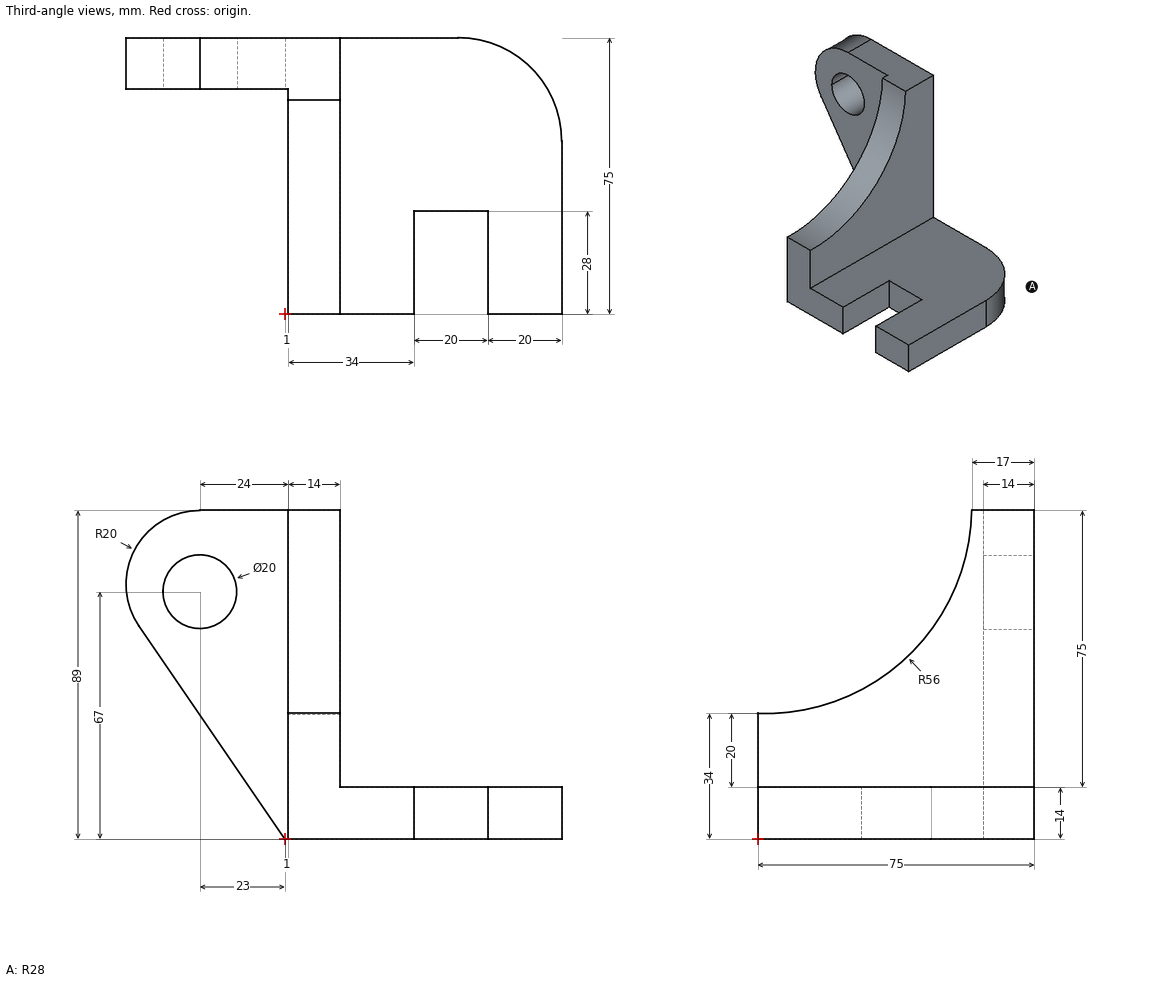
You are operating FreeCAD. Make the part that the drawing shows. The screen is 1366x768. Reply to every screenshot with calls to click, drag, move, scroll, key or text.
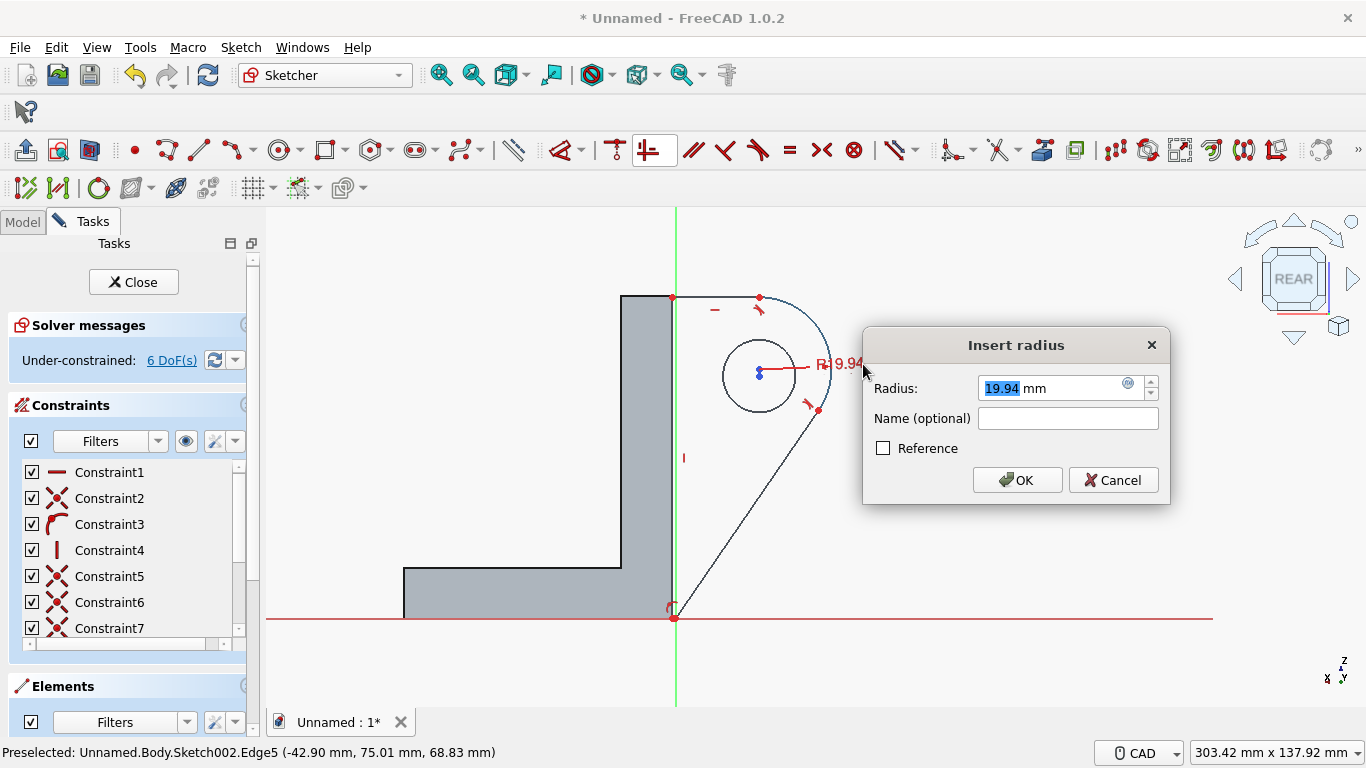
text(20)
key(Return)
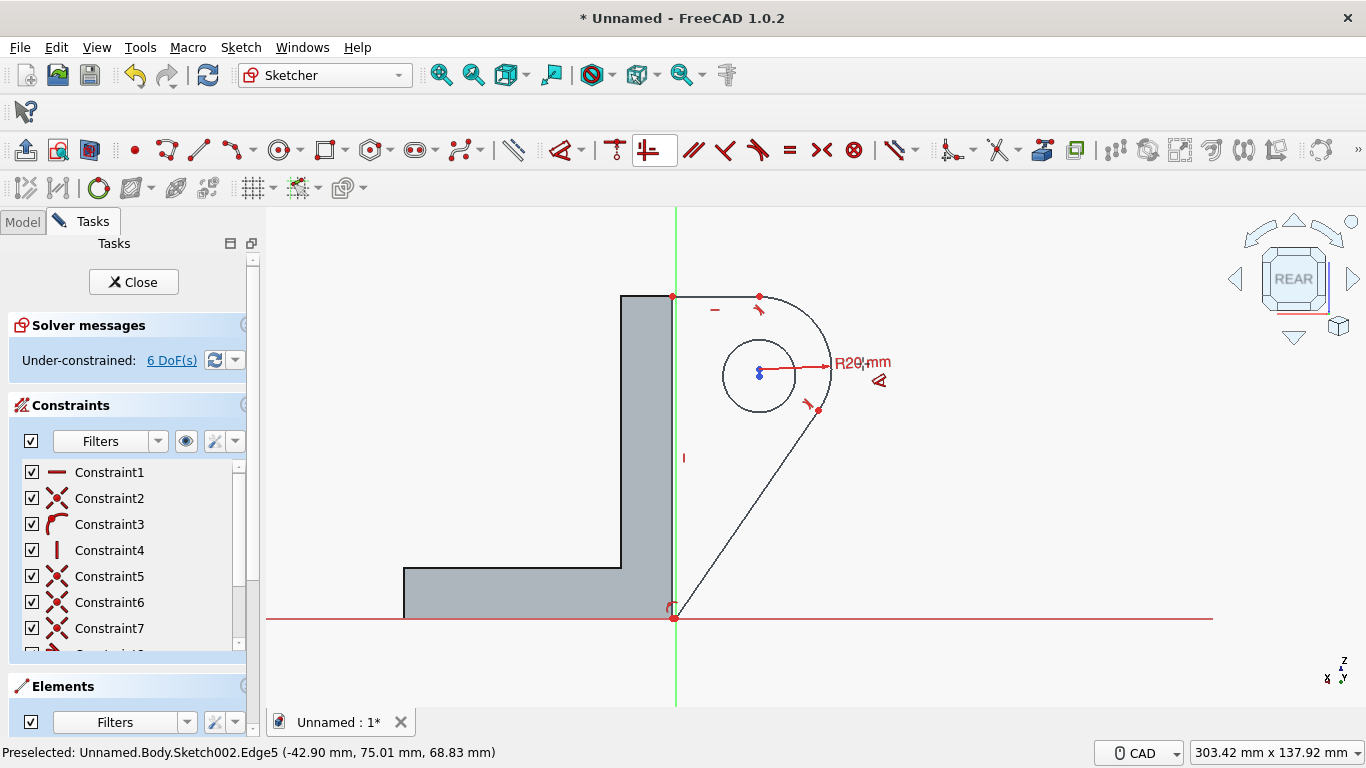
click(785, 350)
click(710, 328)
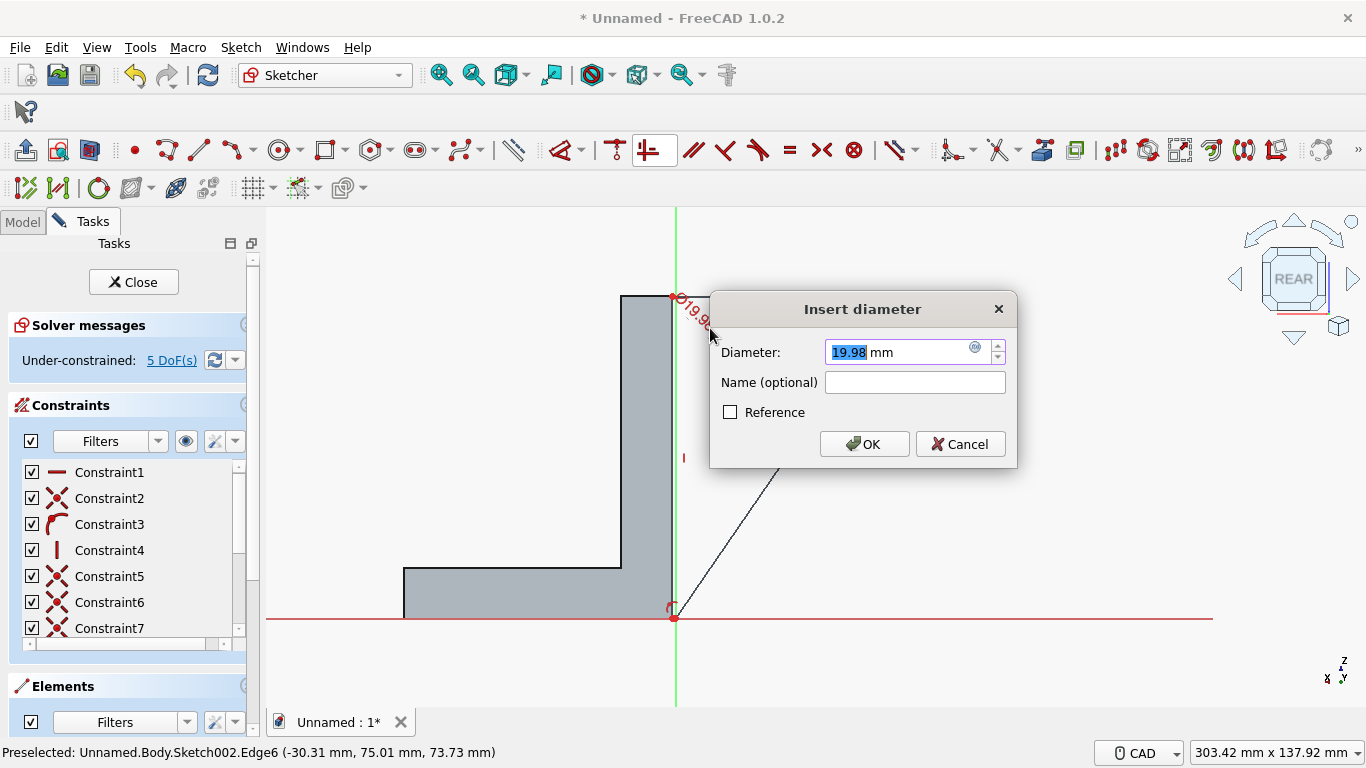
text(20)
key(Return)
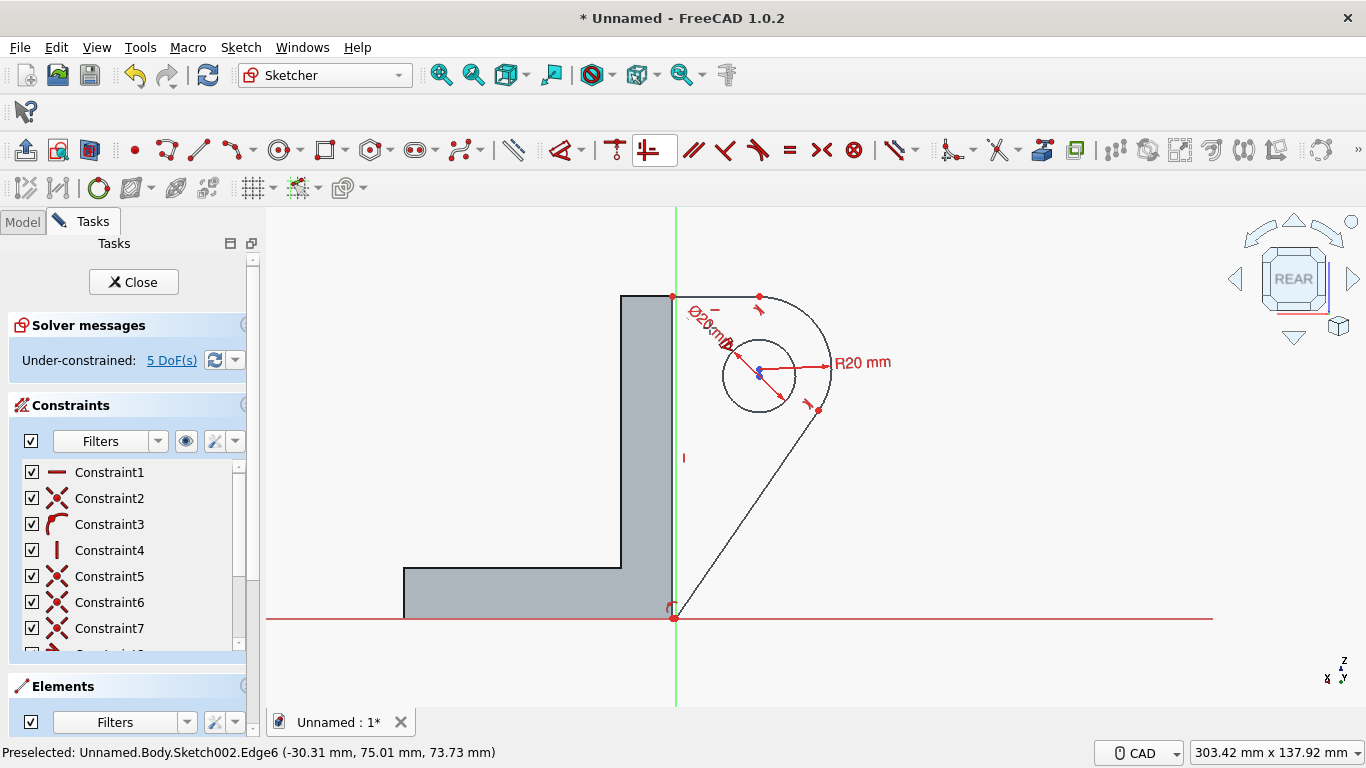
scroll(674, 619, up, 12)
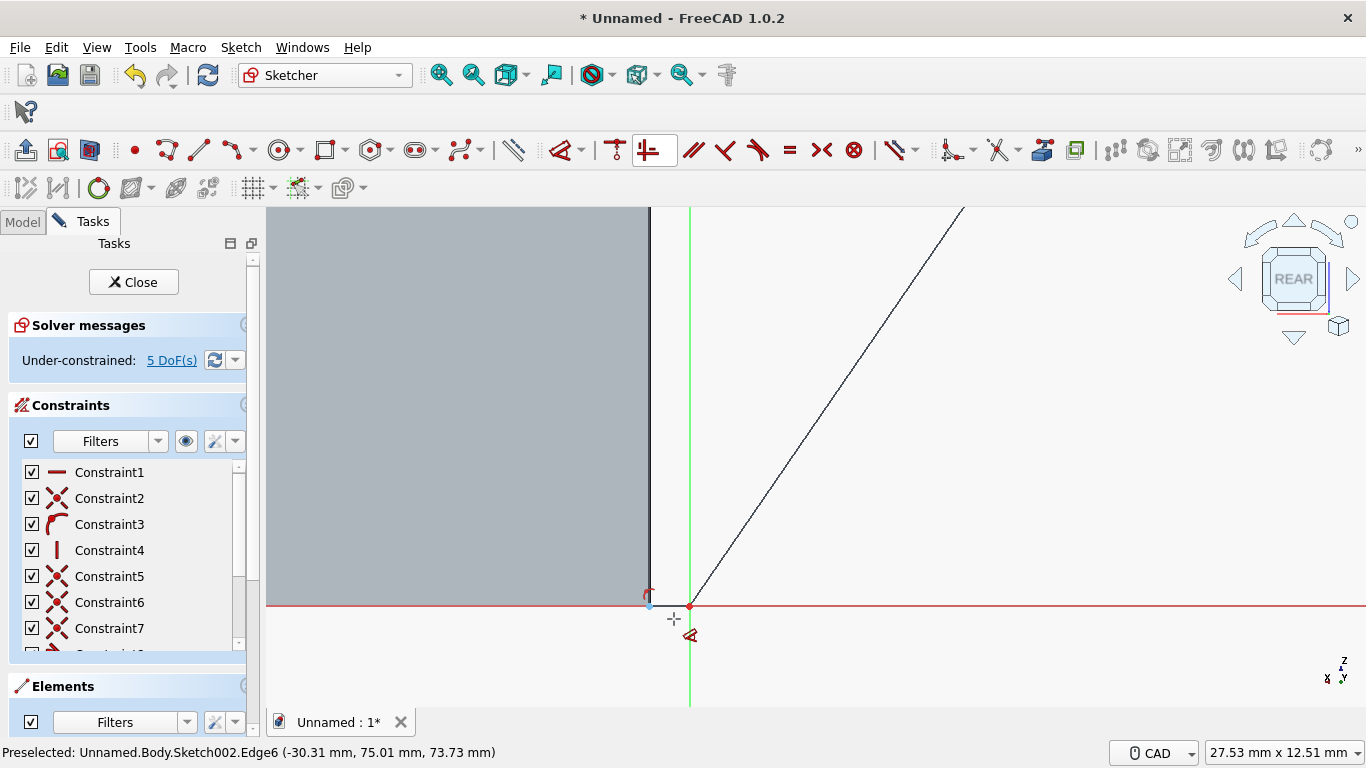
click(670, 606)
click(670, 640)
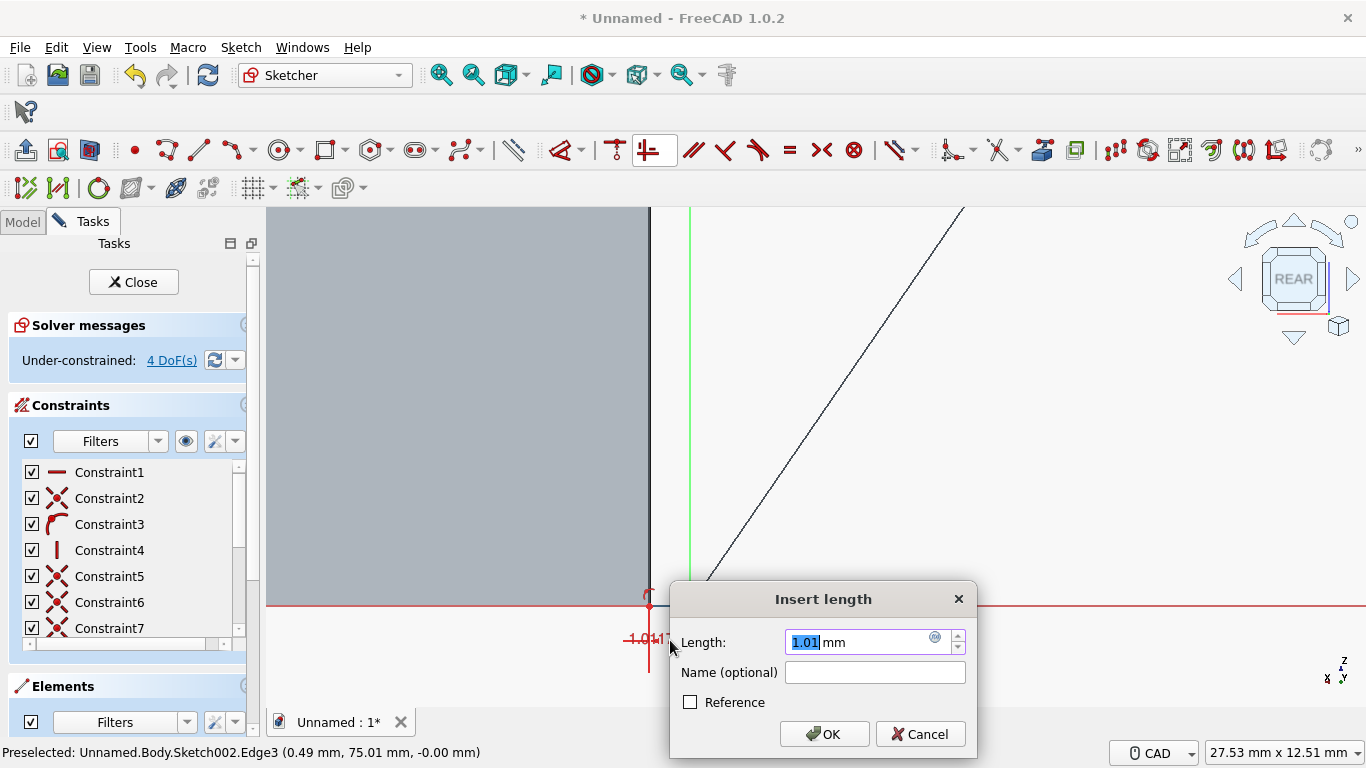
text(1)
key(Return)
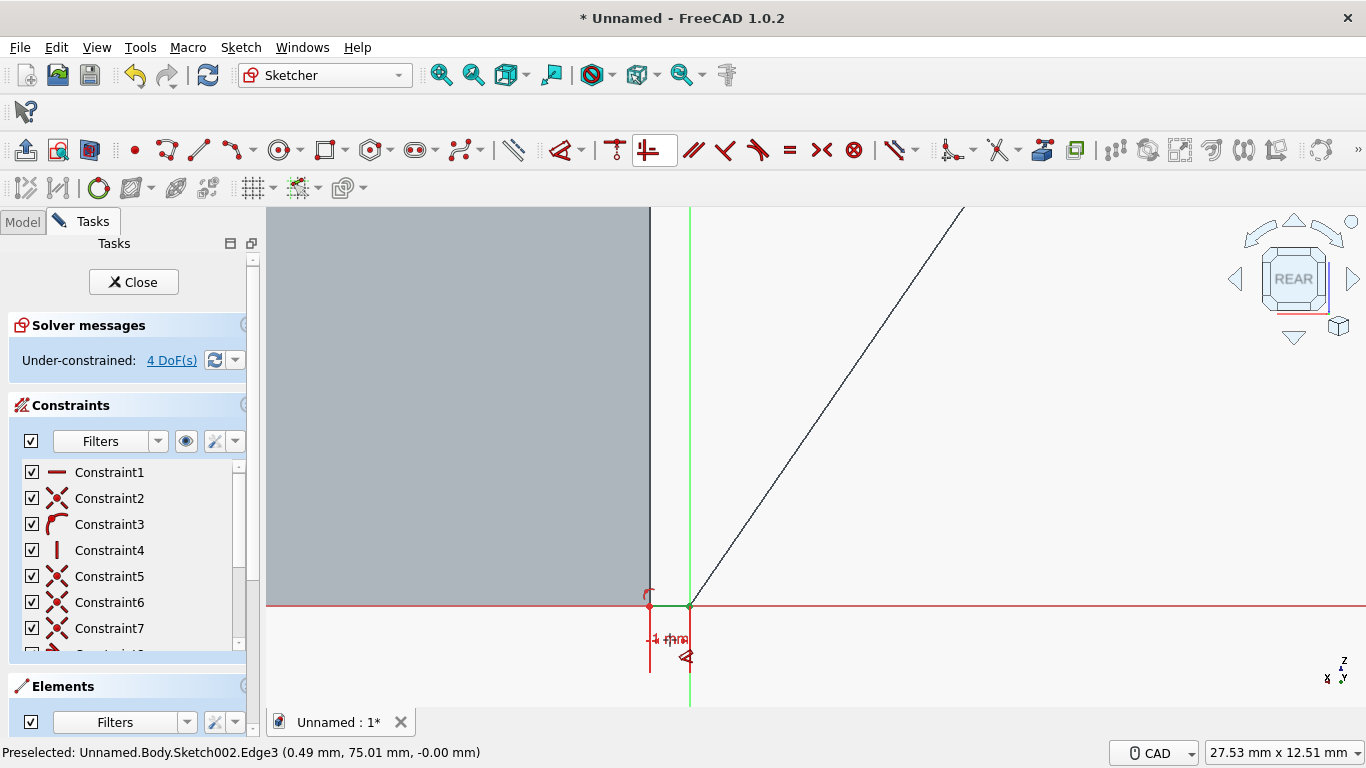
scroll(674, 620, down, 12)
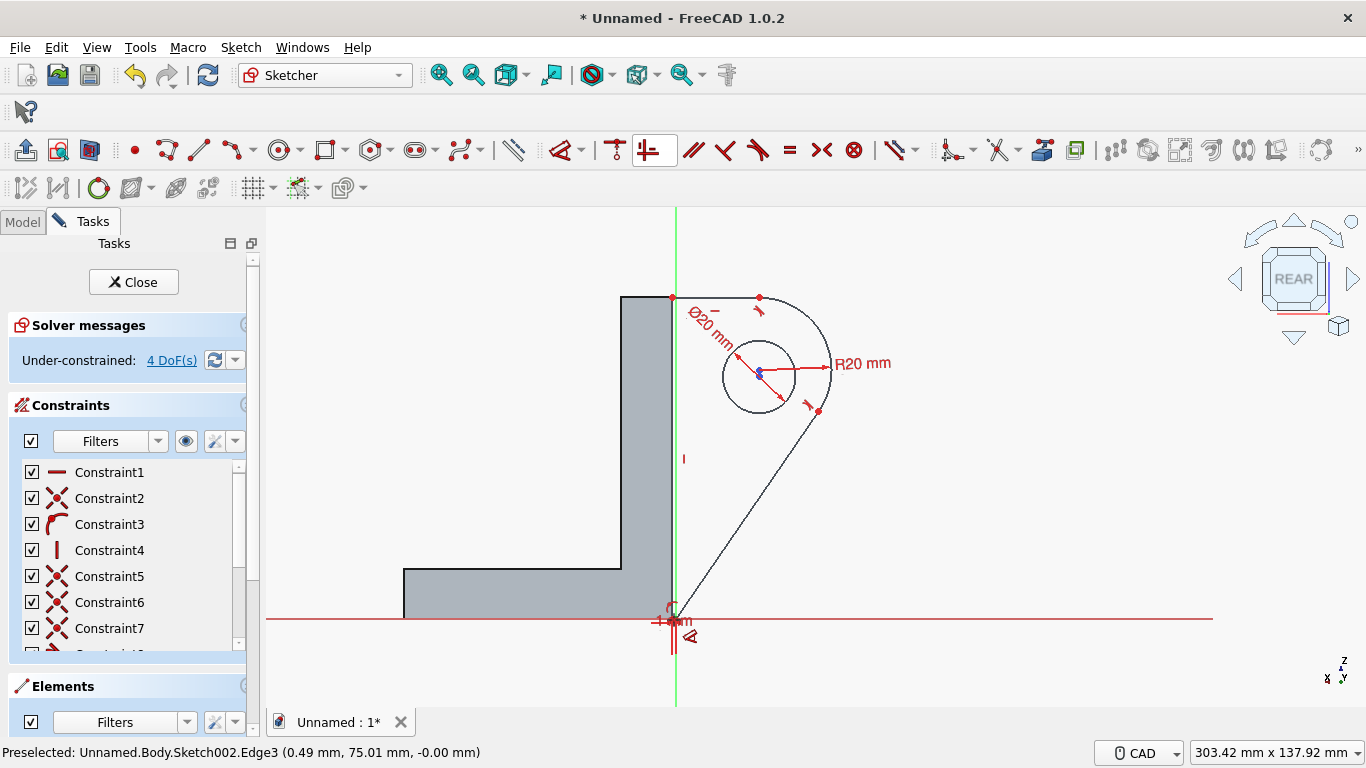
click(733, 298)
click(716, 264)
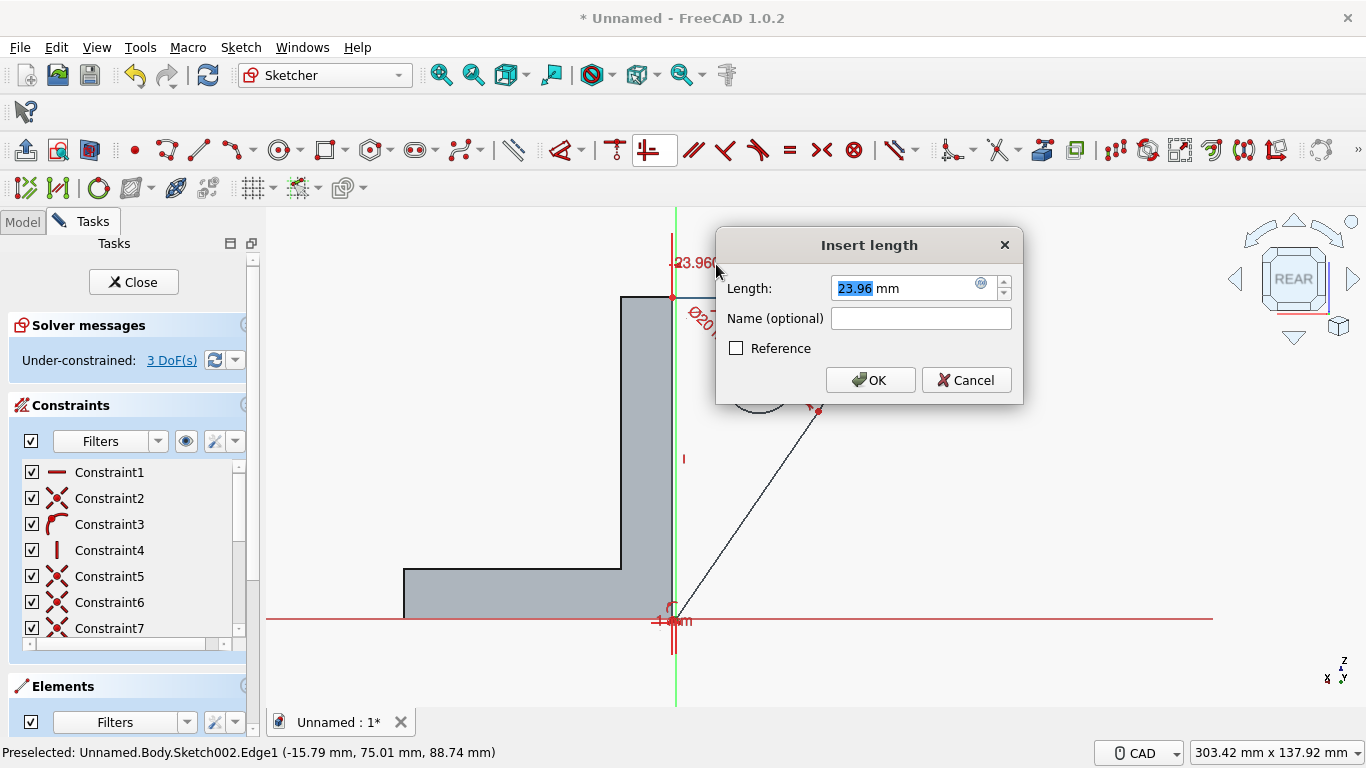
text(24)
key(Return)